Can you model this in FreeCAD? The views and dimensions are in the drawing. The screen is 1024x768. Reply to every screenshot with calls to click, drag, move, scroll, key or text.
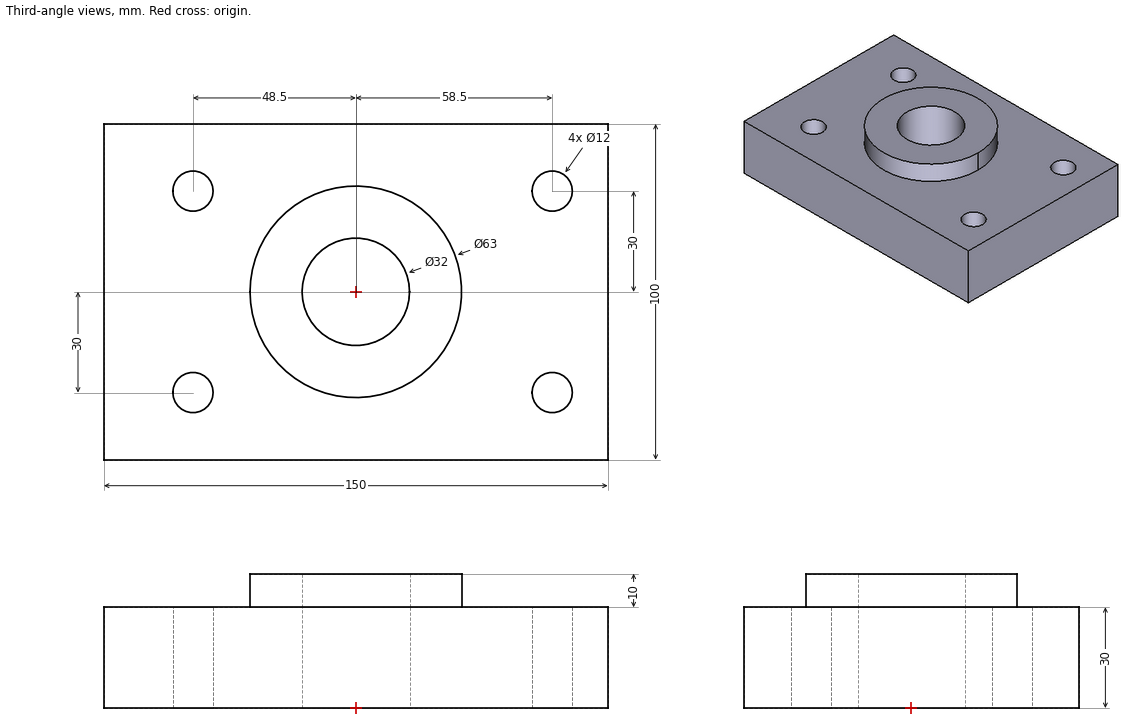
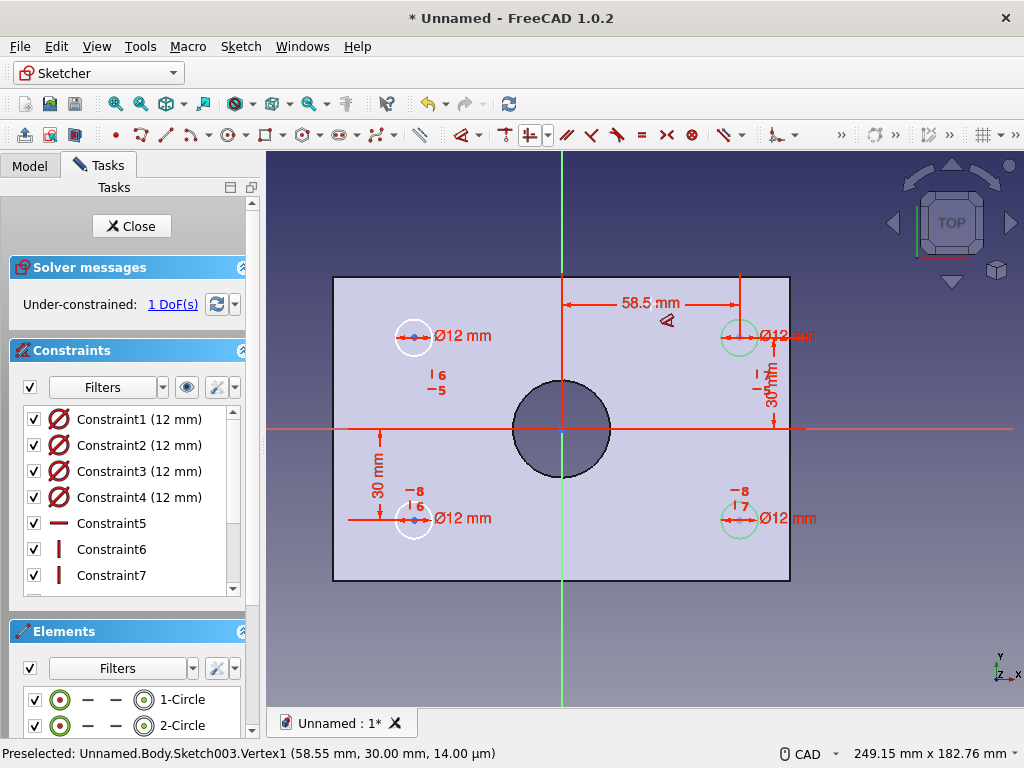
click(414, 338)
click(488, 304)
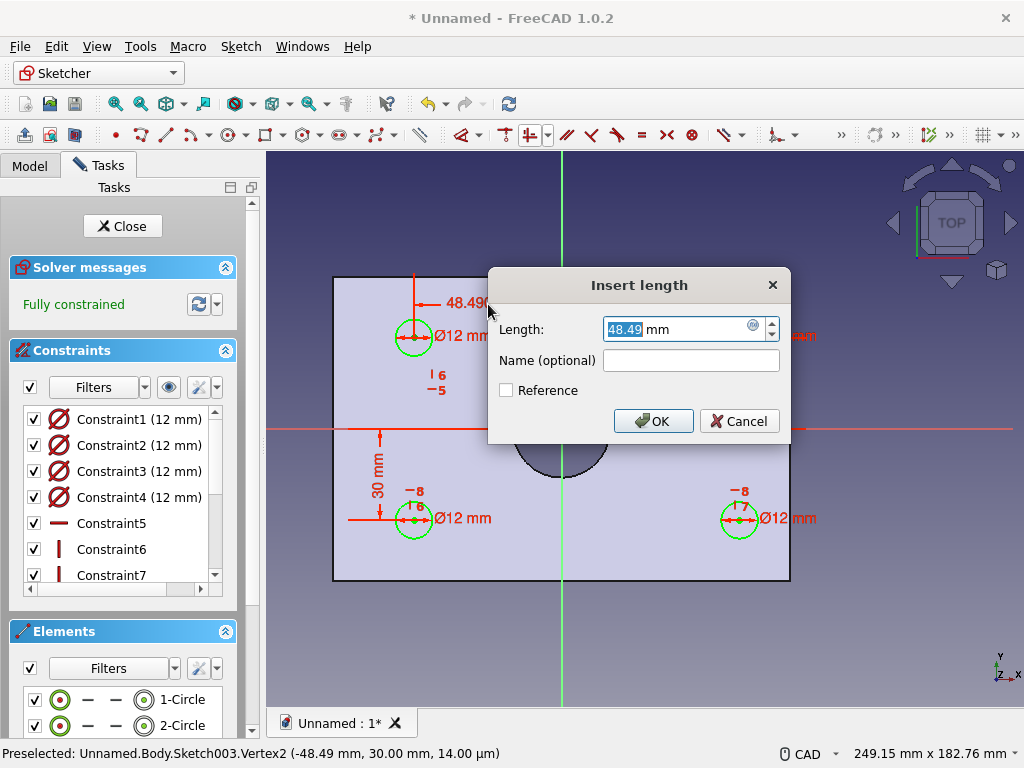
text(48.5)
key(Return)
key(Escape)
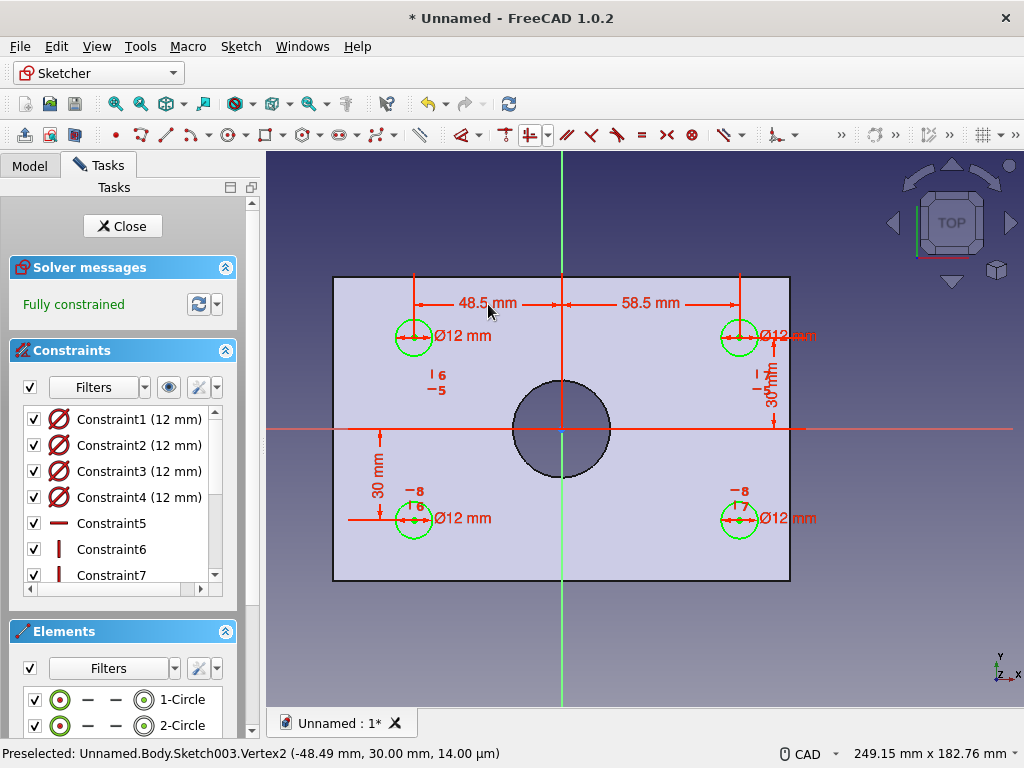
click(123, 226)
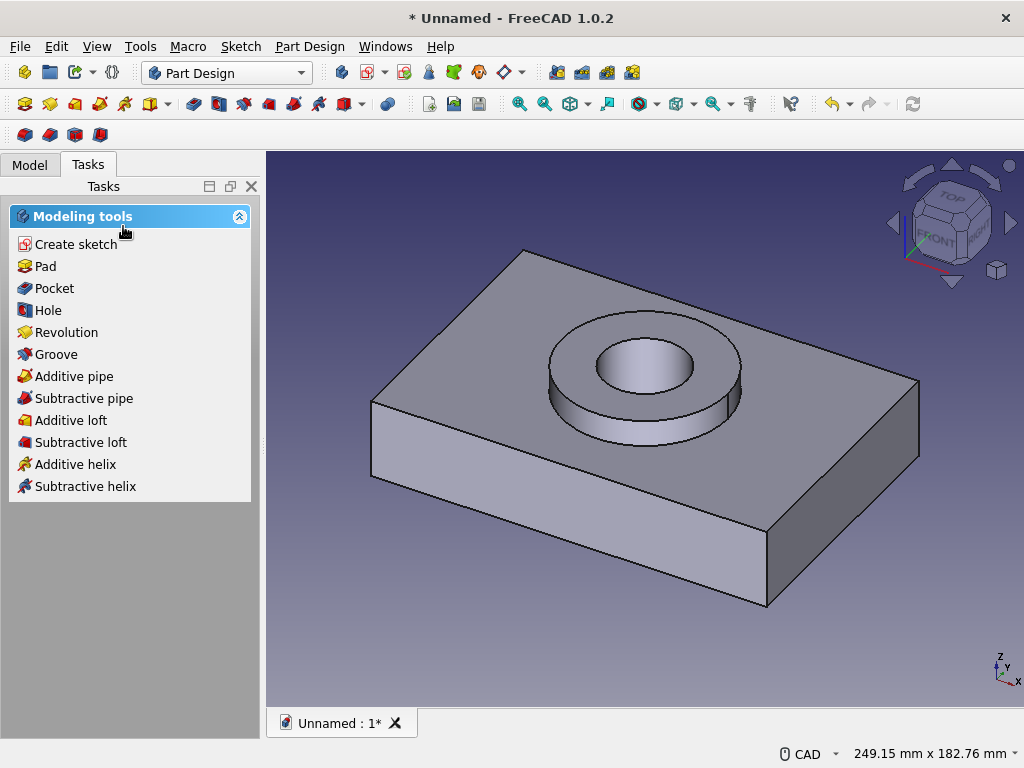
click(194, 104)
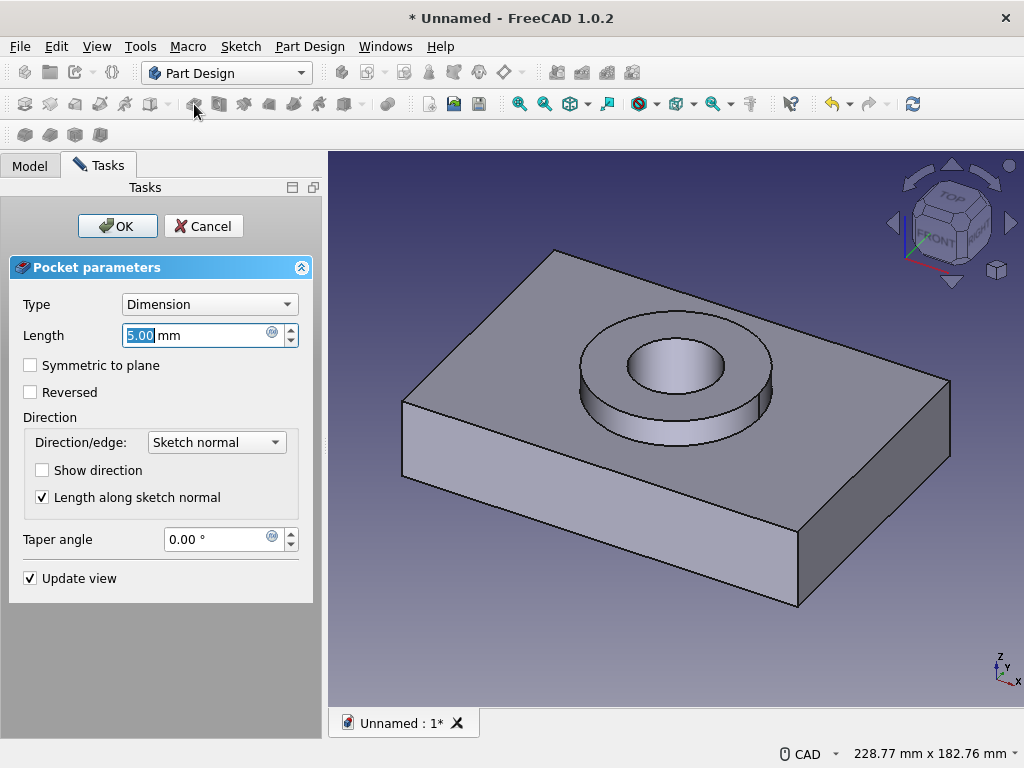
click(210, 304)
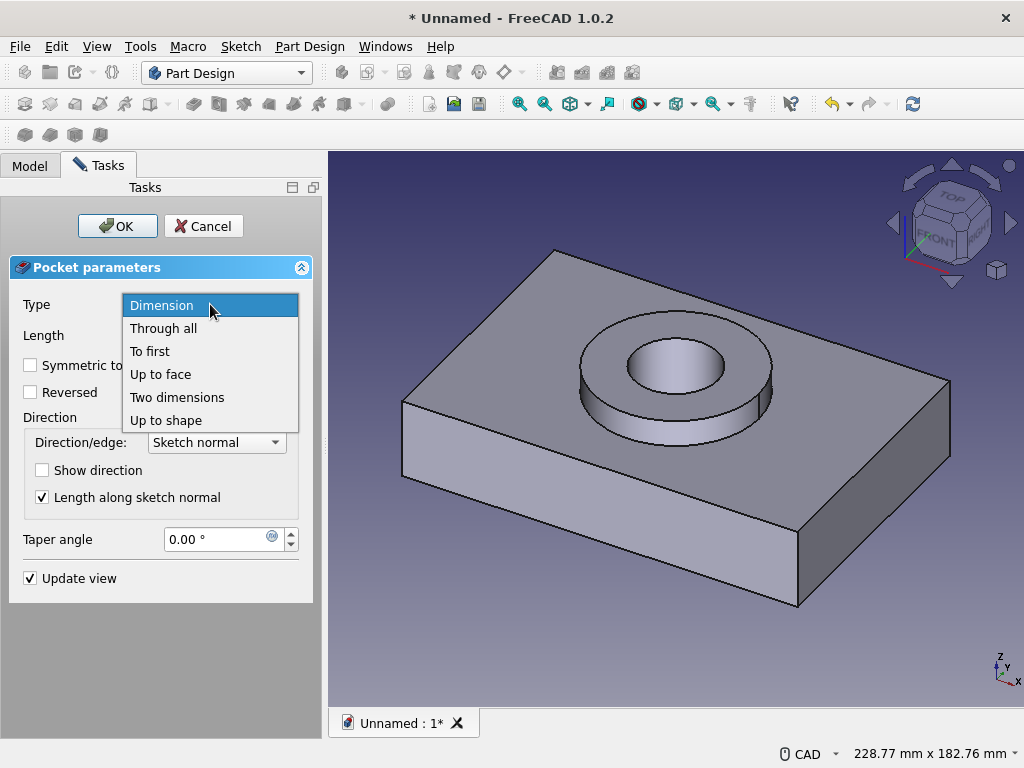
click(208, 328)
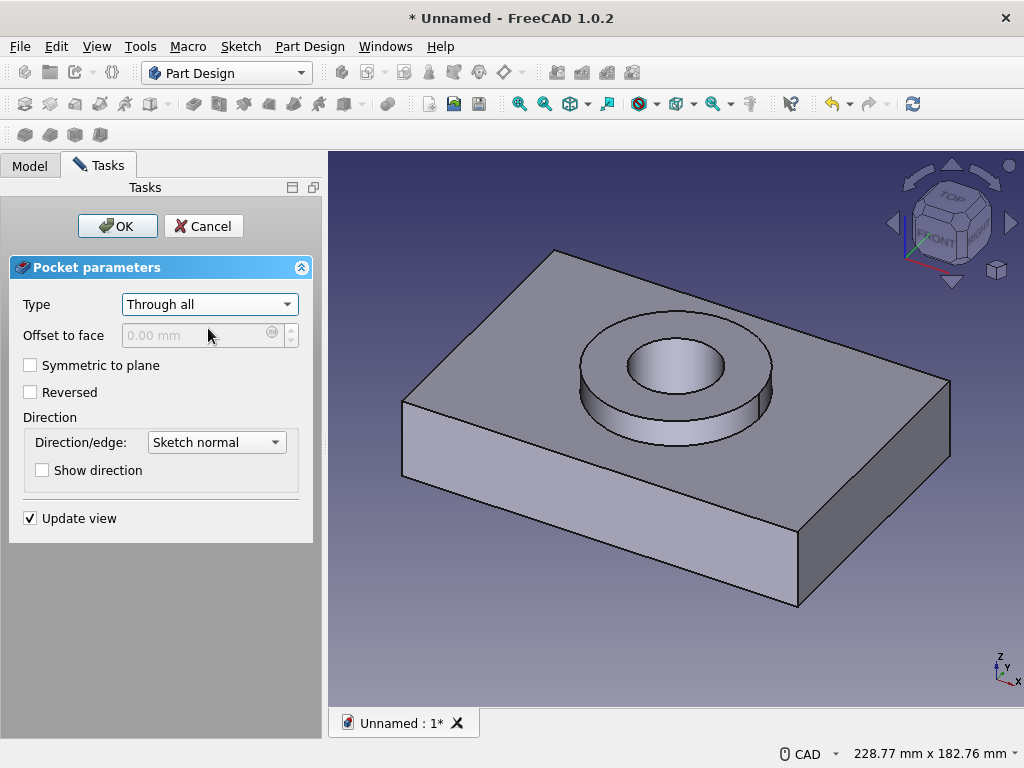
click(31, 392)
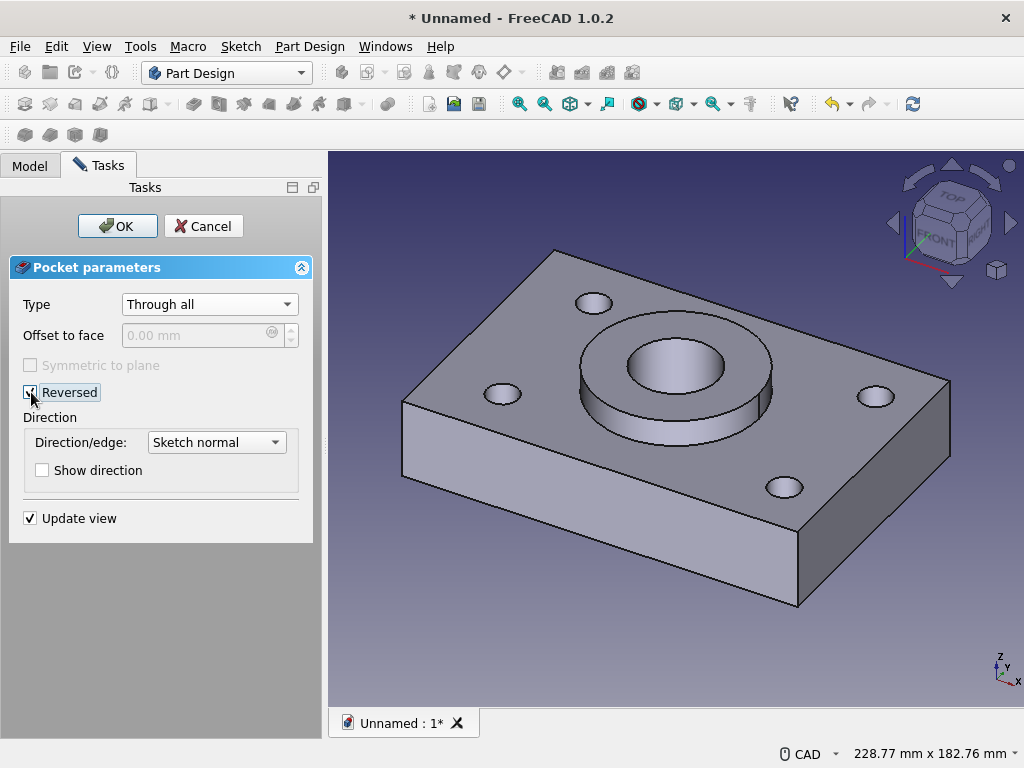
click(118, 226)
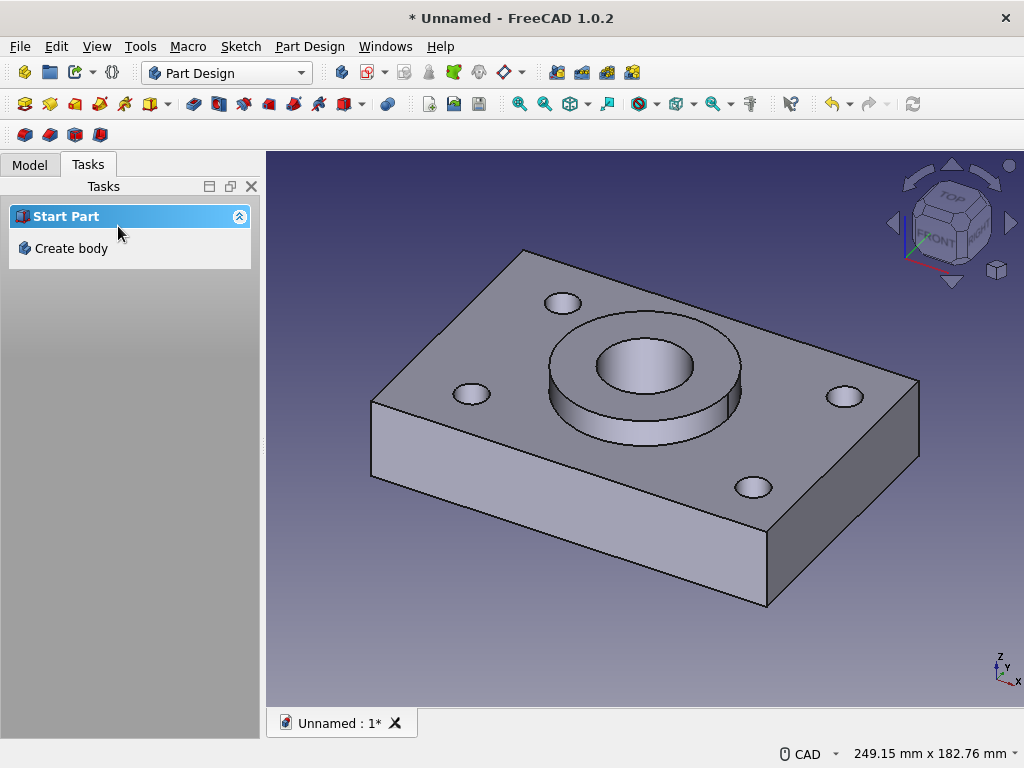
key(0)